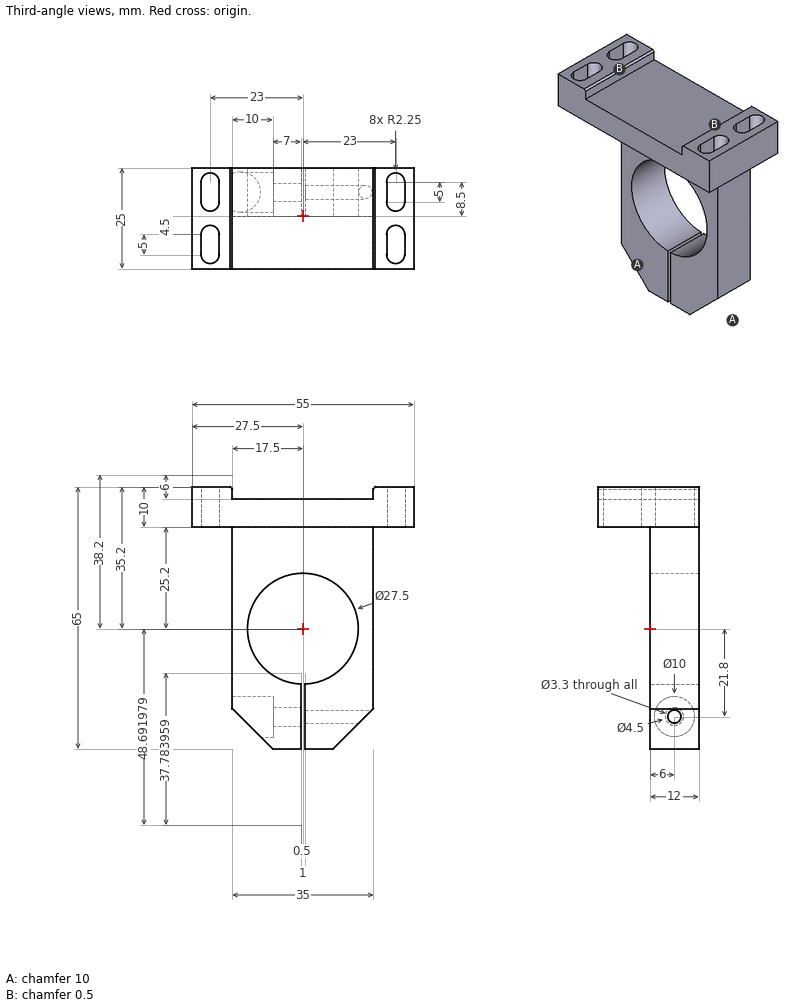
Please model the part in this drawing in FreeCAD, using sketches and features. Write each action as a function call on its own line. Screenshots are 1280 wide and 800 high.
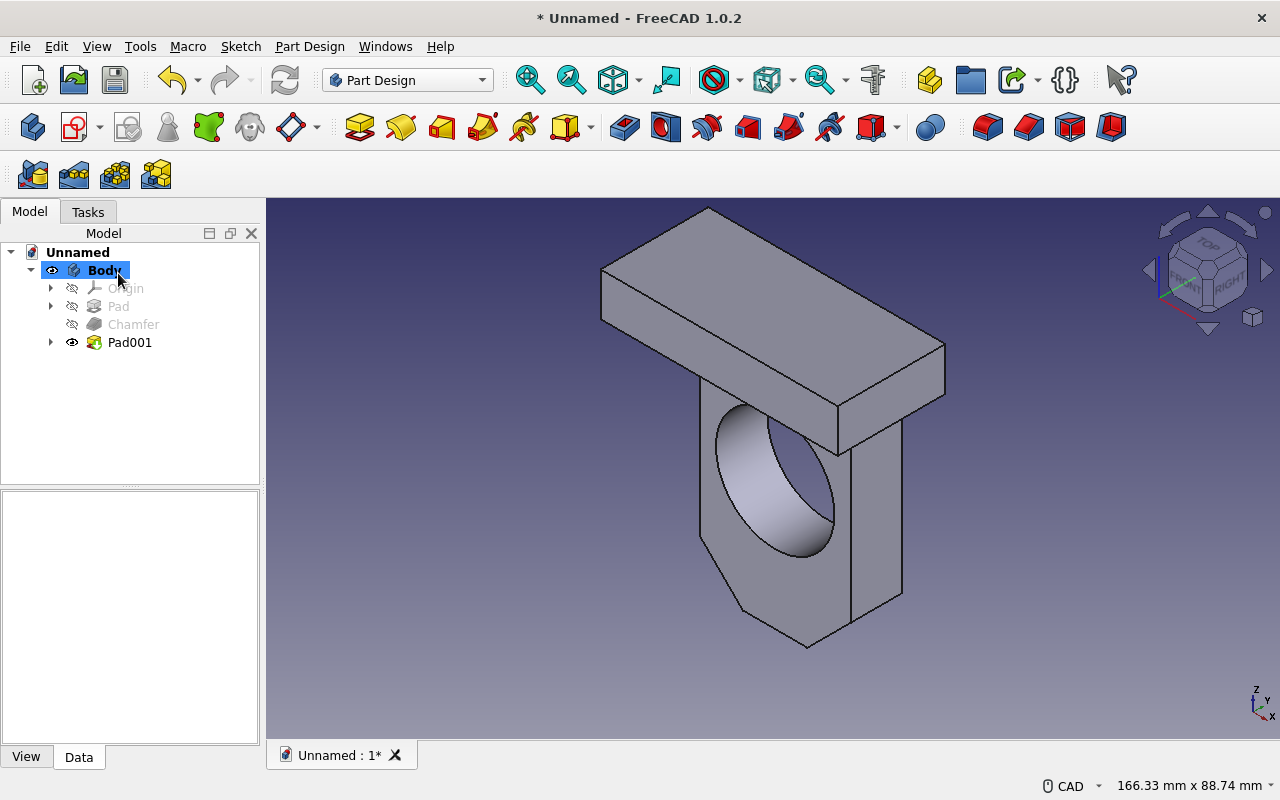
click(787, 401)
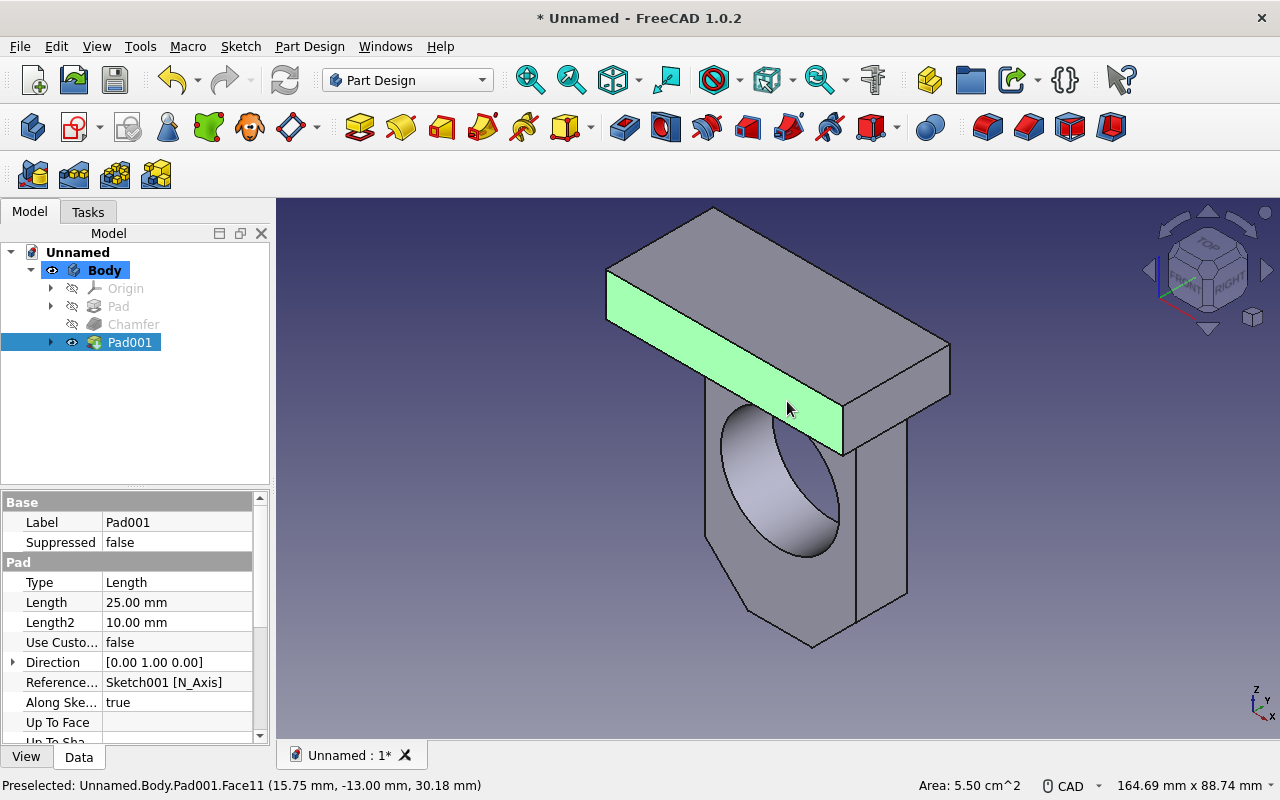
click(74, 128)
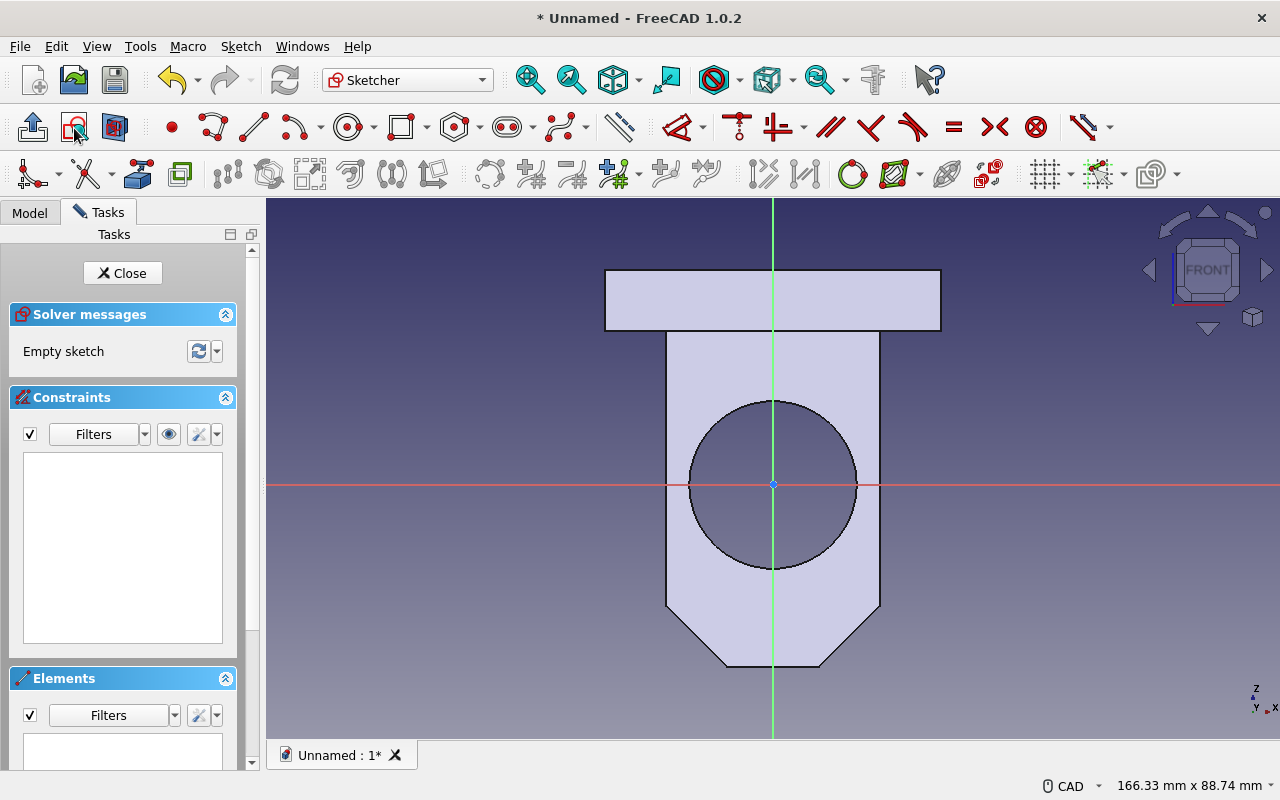
scroll(912, 226, up, 2)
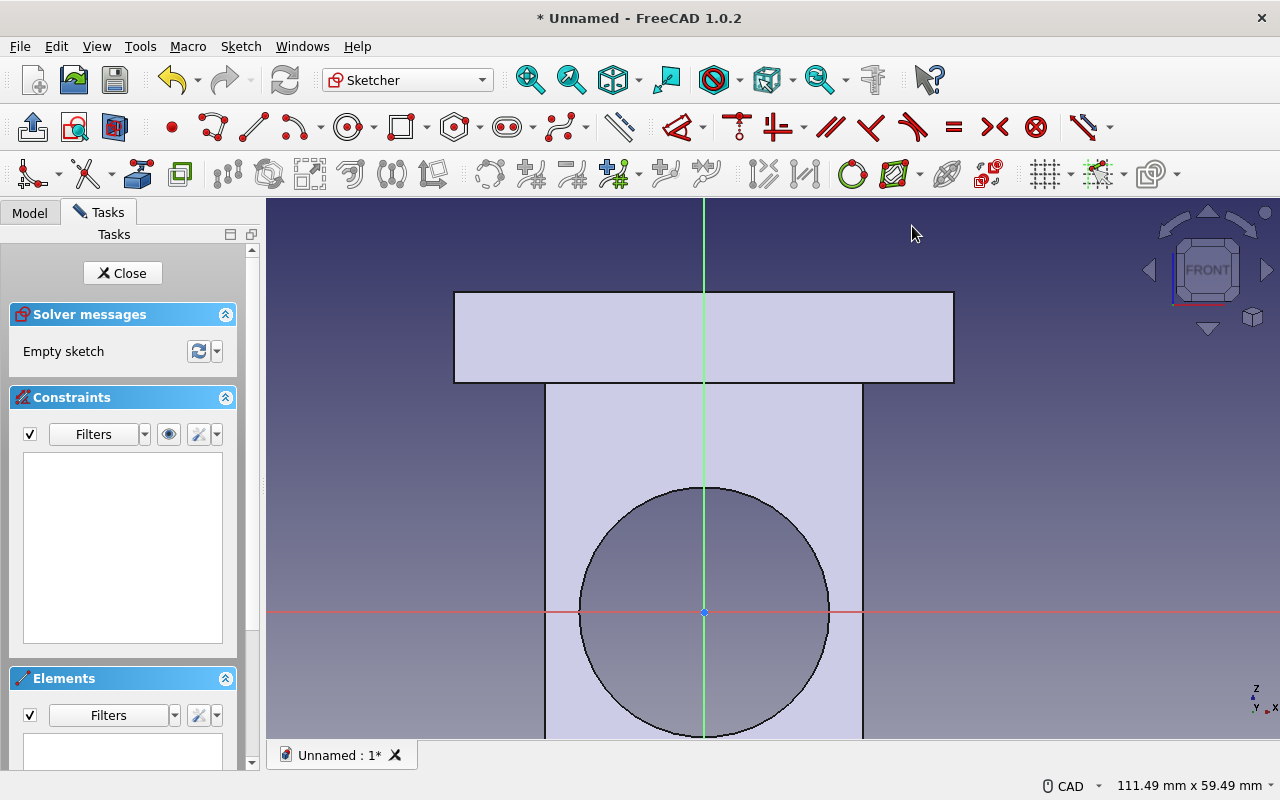
click(400, 128)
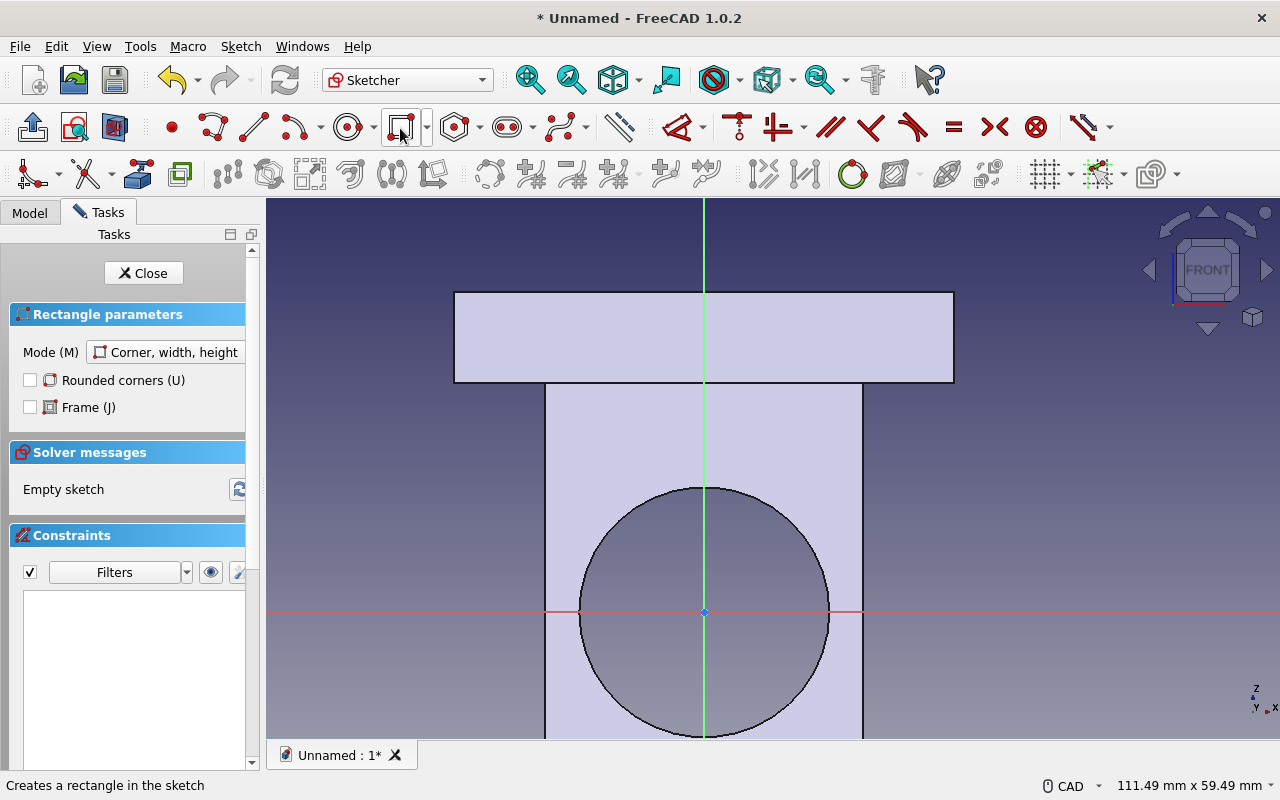
click(545, 265)
click(863, 319)
key(Escape)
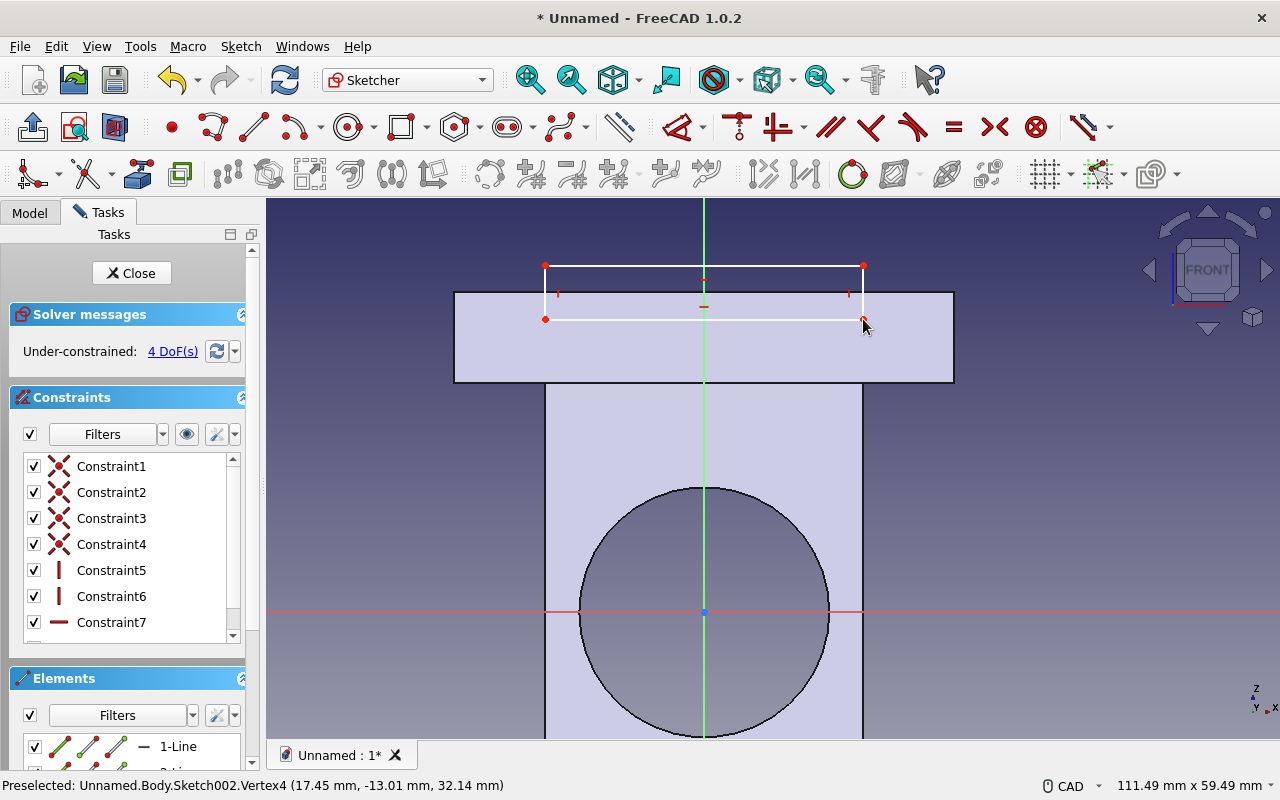
click(676, 128)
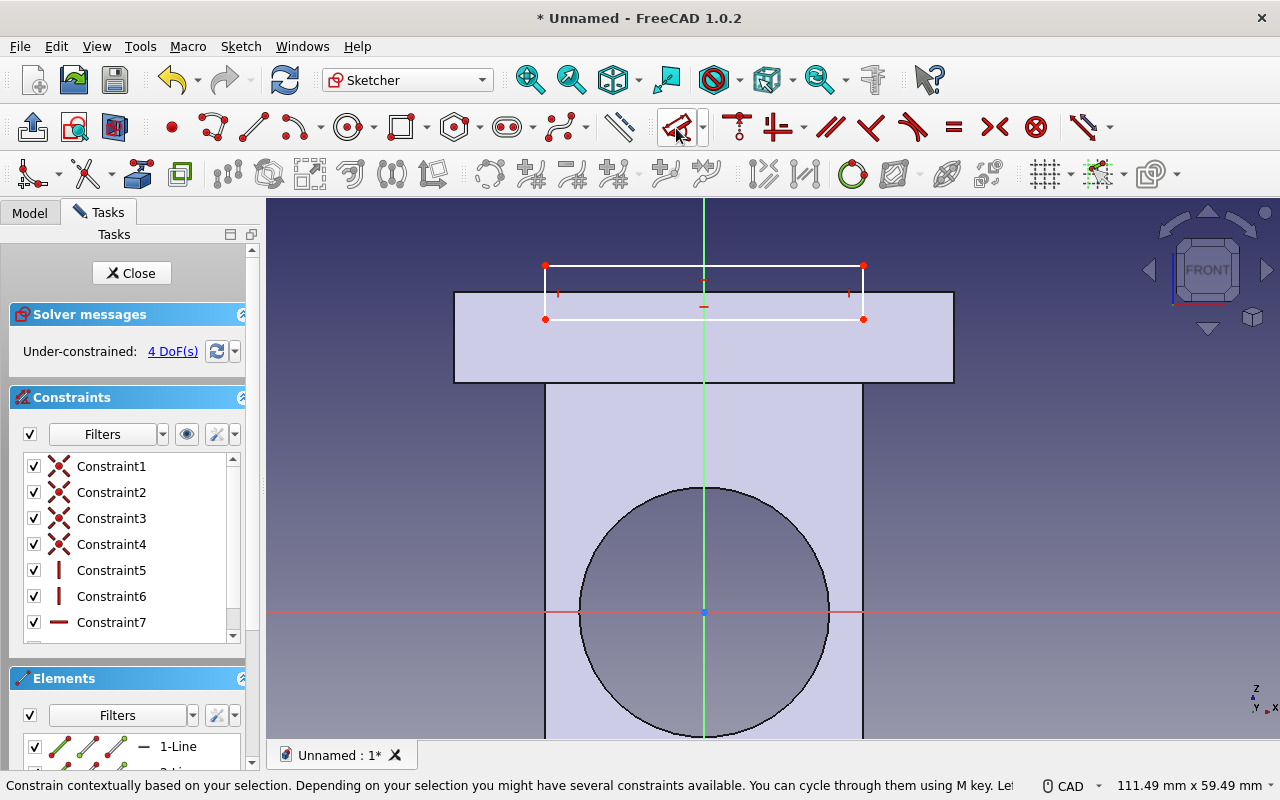
click(545, 282)
click(511, 293)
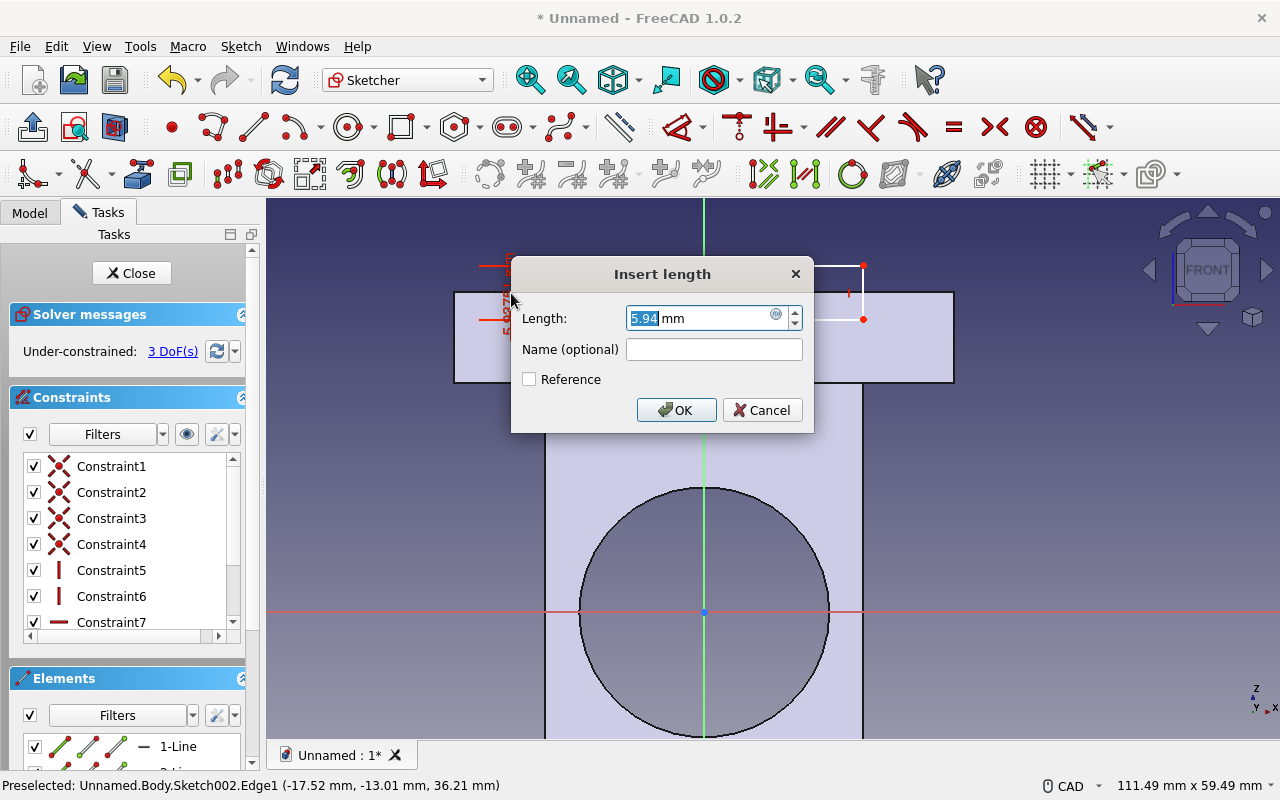
text(6)
key(Return)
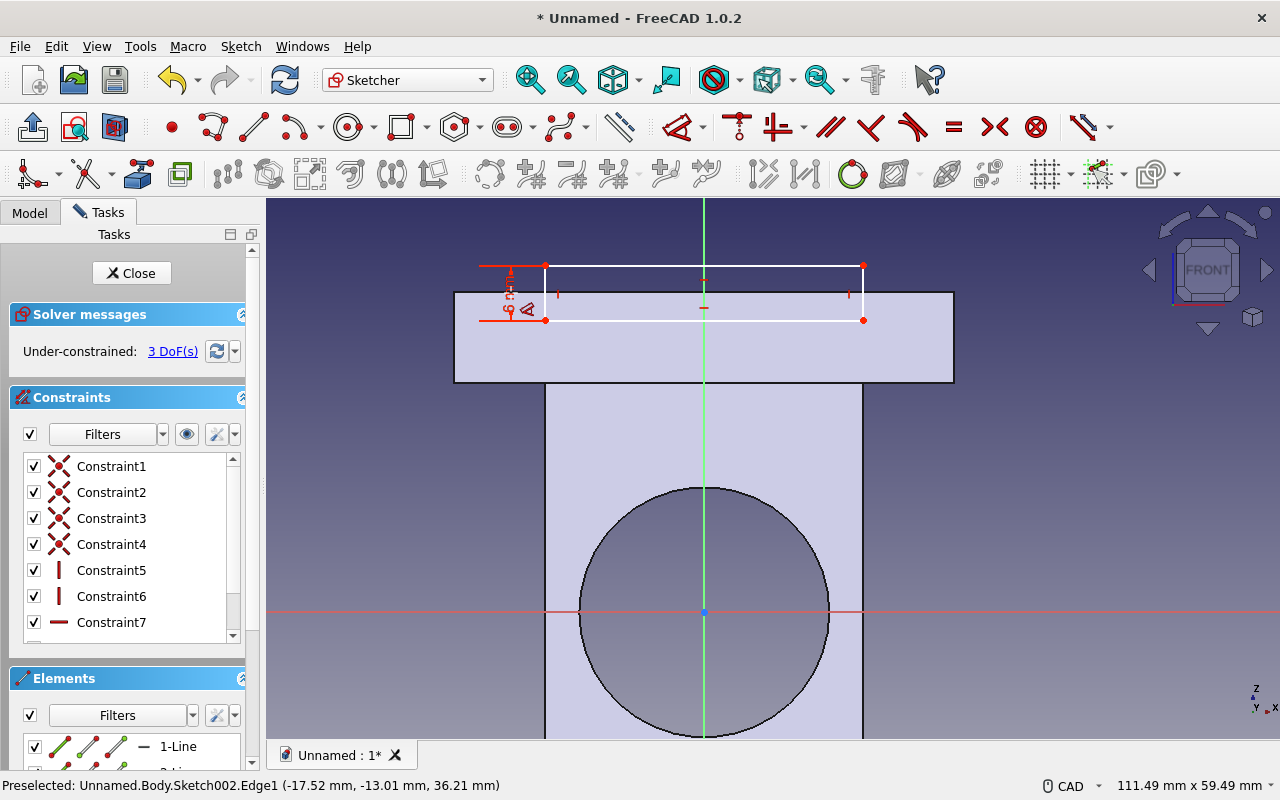
click(640, 321)
click(631, 287)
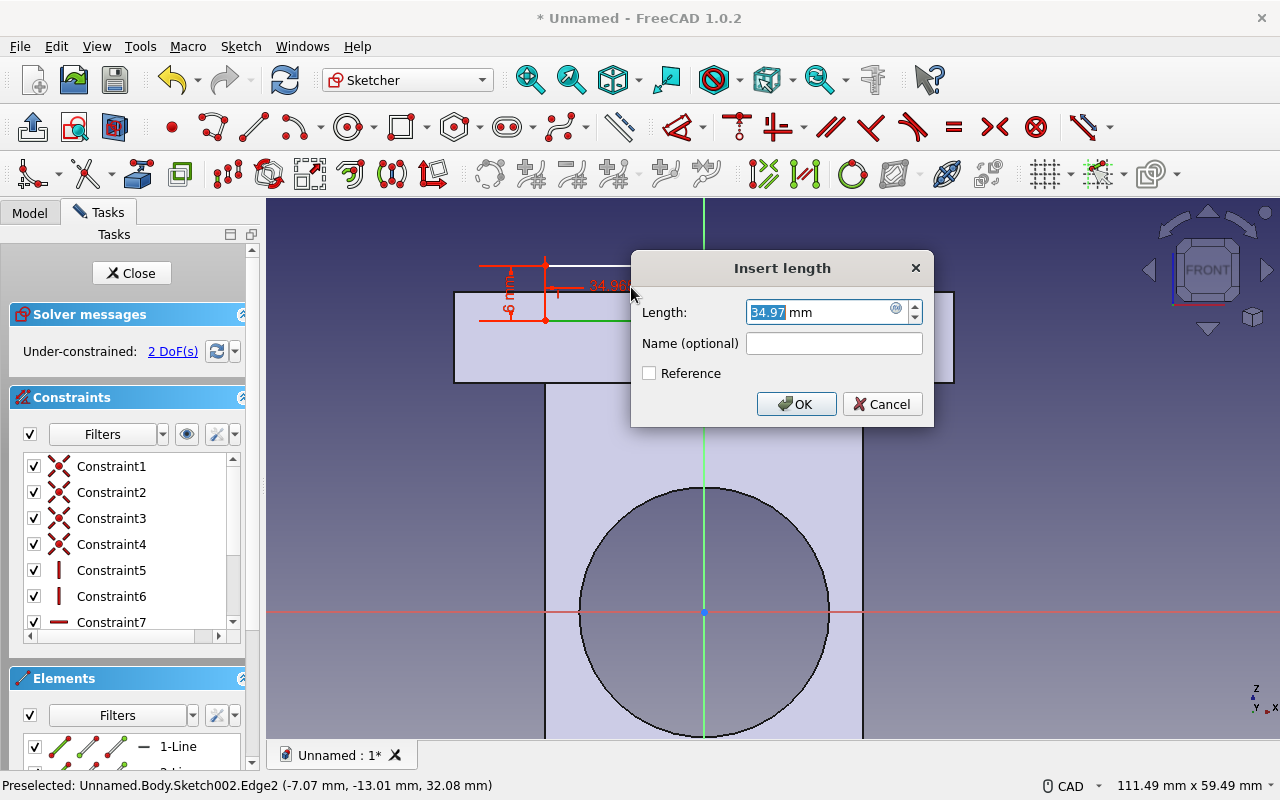
text(35)
key(Return)